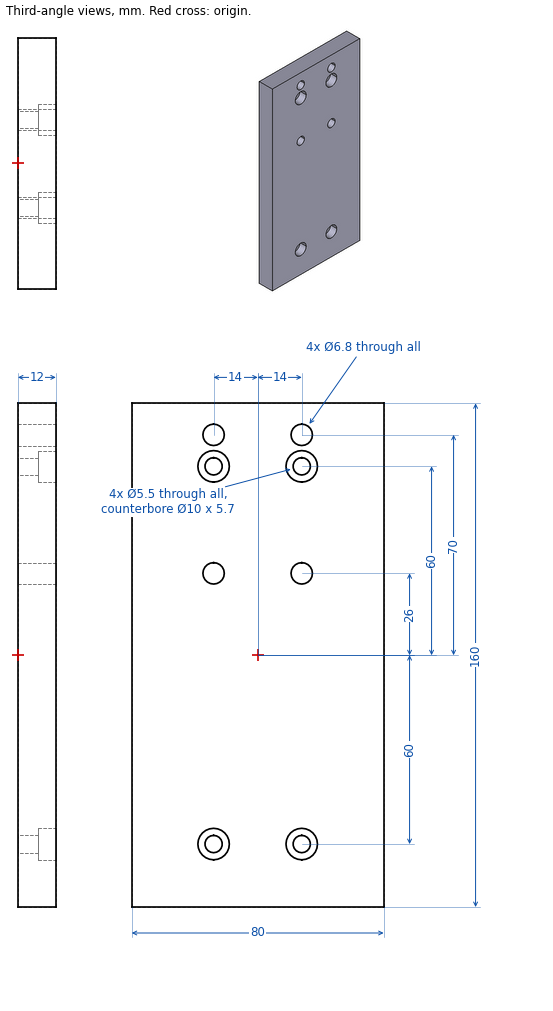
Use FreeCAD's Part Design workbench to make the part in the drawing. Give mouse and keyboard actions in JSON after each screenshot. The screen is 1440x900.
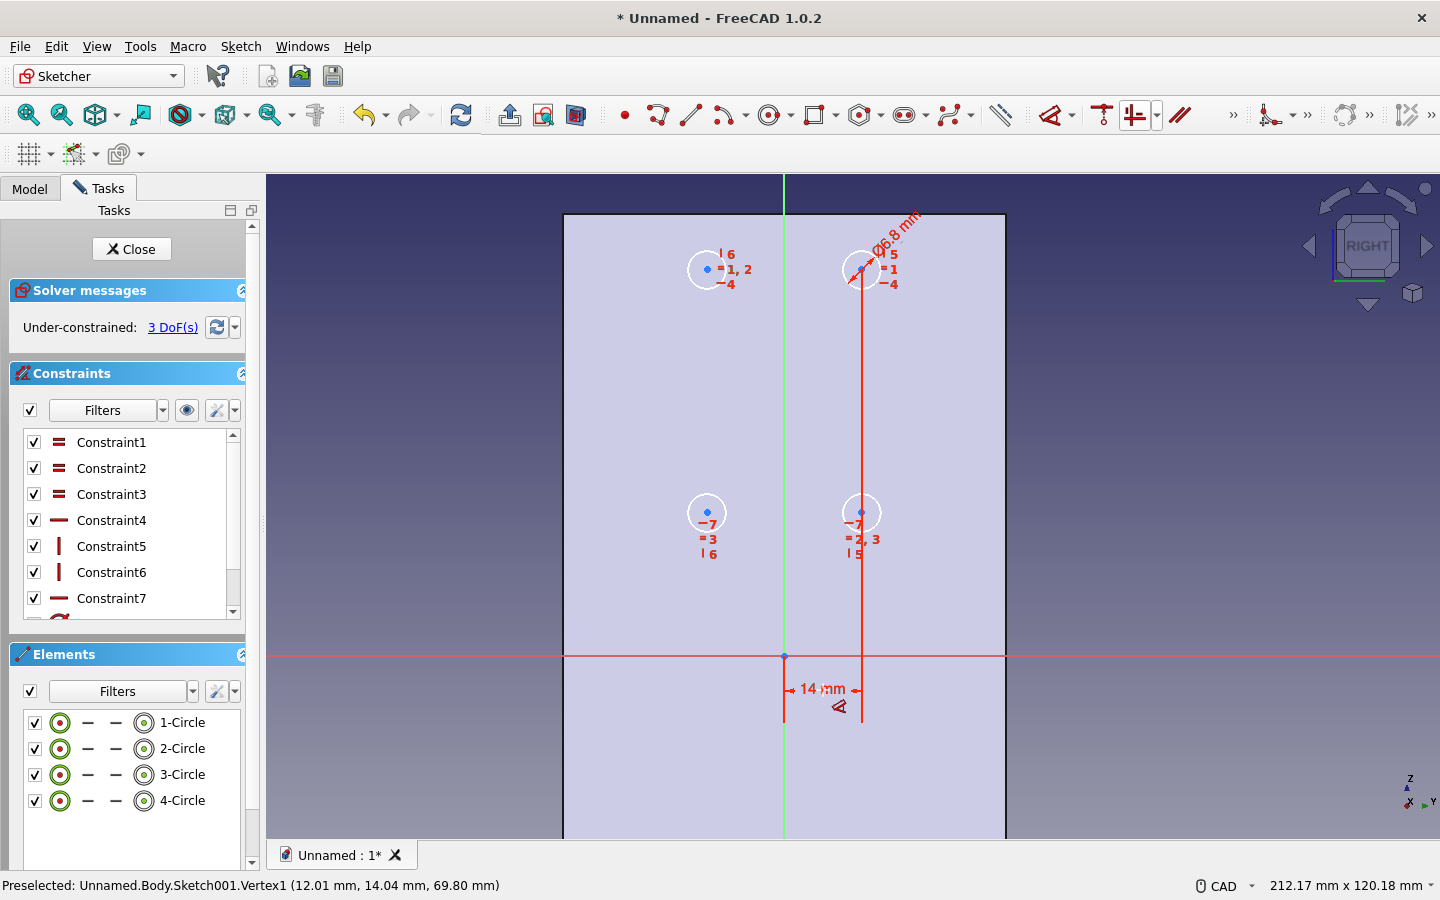
{"action": "left_click", "coordinate": [862, 270]}
{"action": "left_click", "coordinate": [896, 463]}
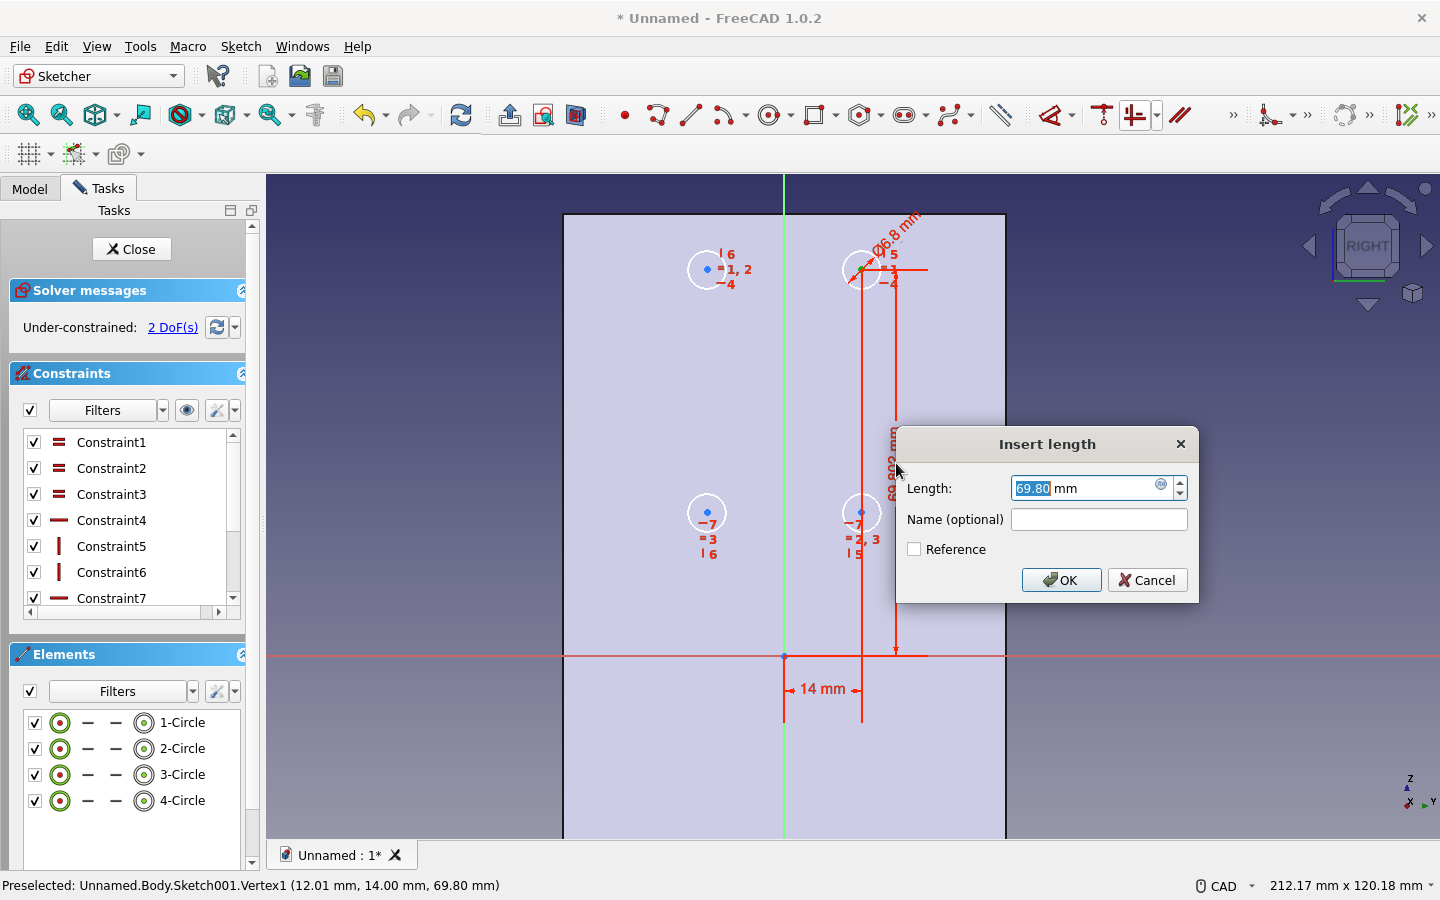
{"action": "type", "text": "70"}
{"action": "key", "text": "Return"}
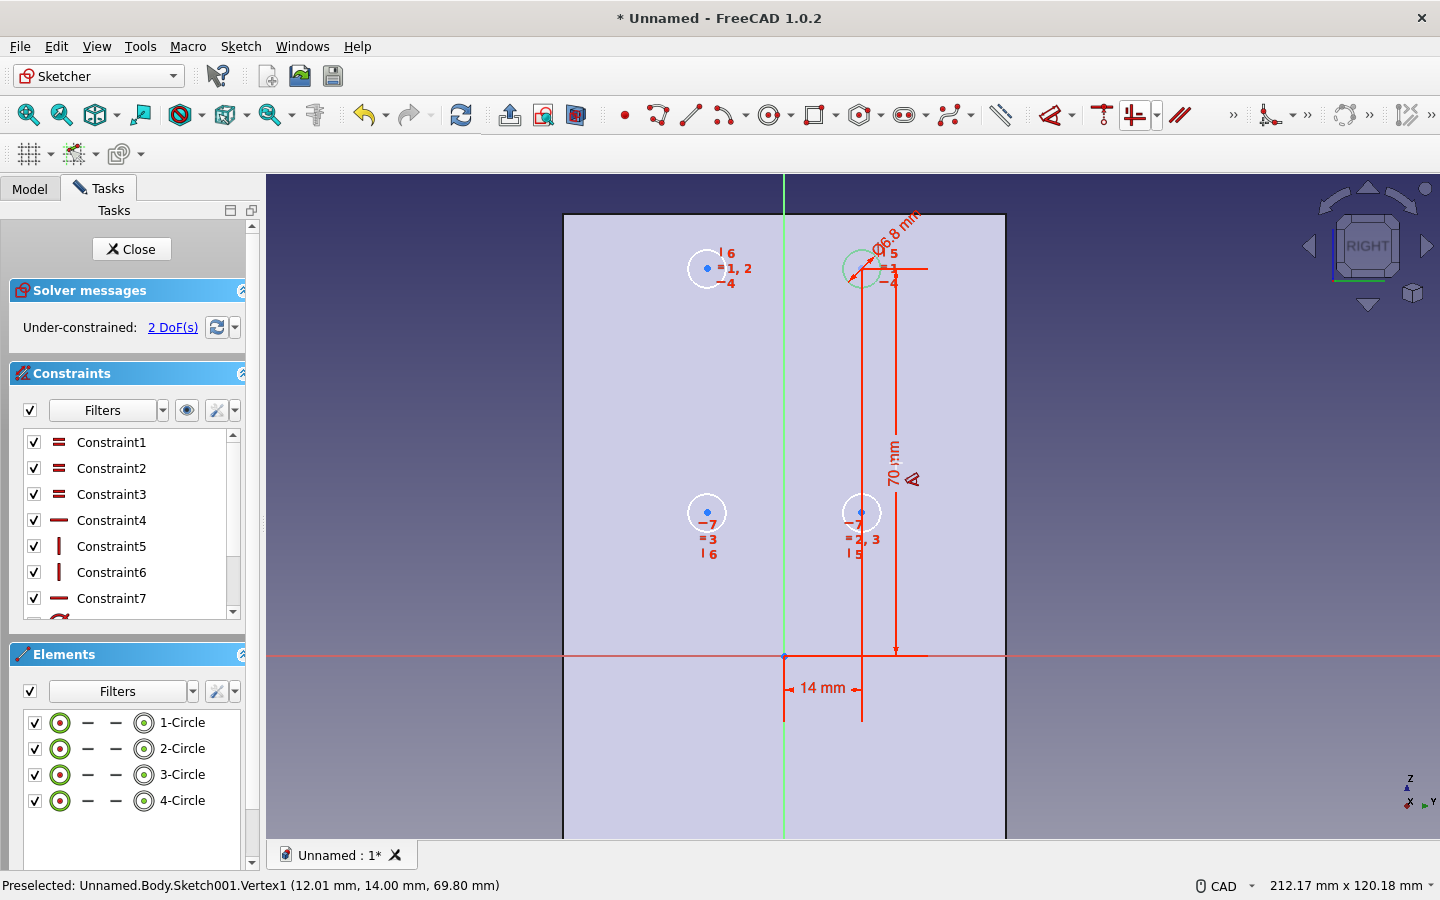
{"action": "left_click", "coordinate": [707, 269]}
{"action": "left_click", "coordinate": [746, 690]}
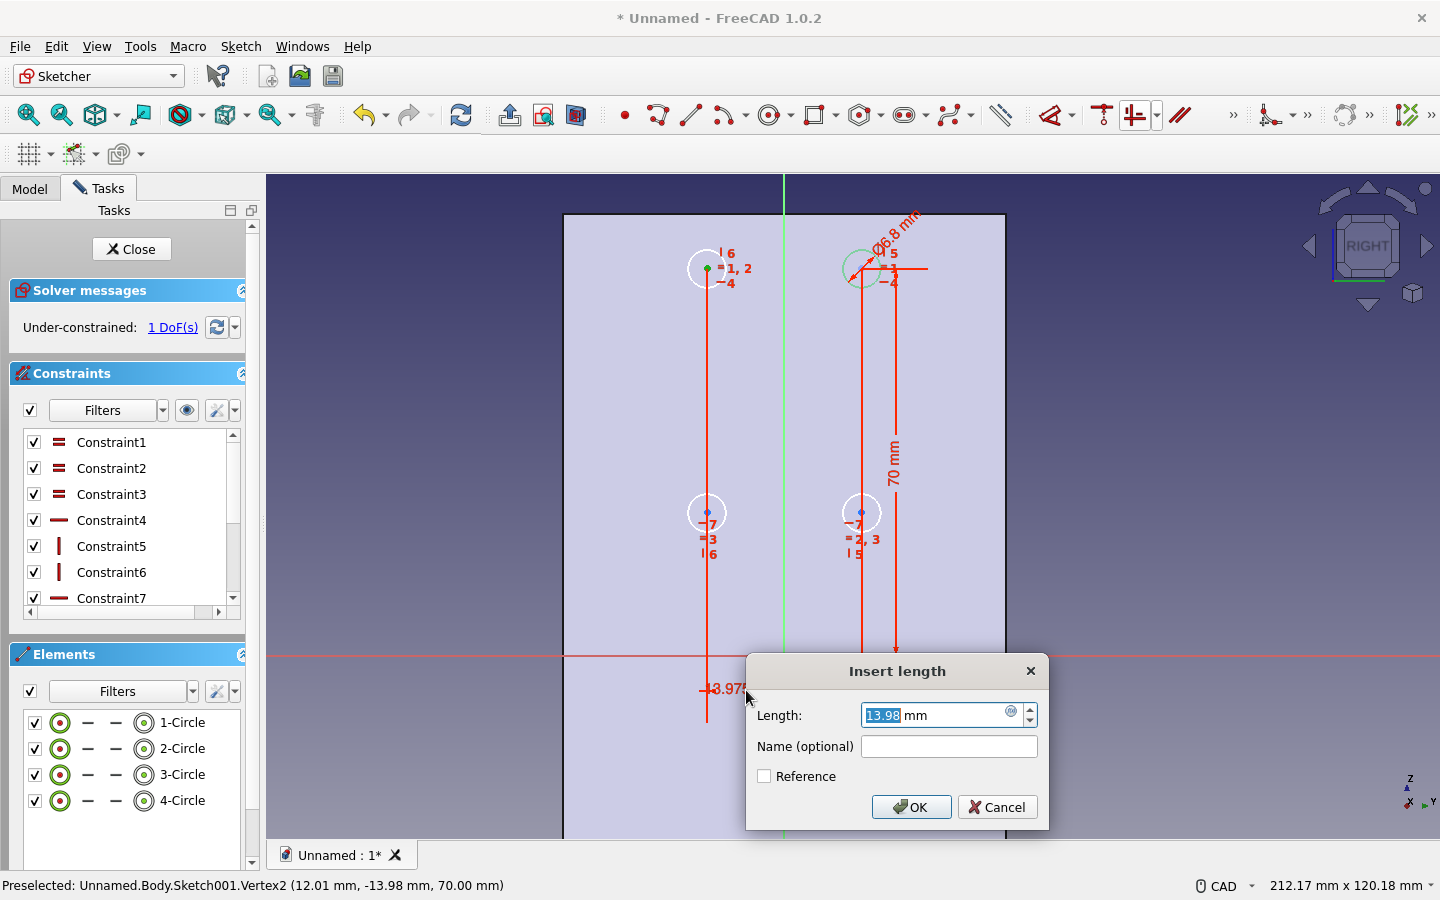
{"action": "type", "text": "14"}
{"action": "key", "text": "Return"}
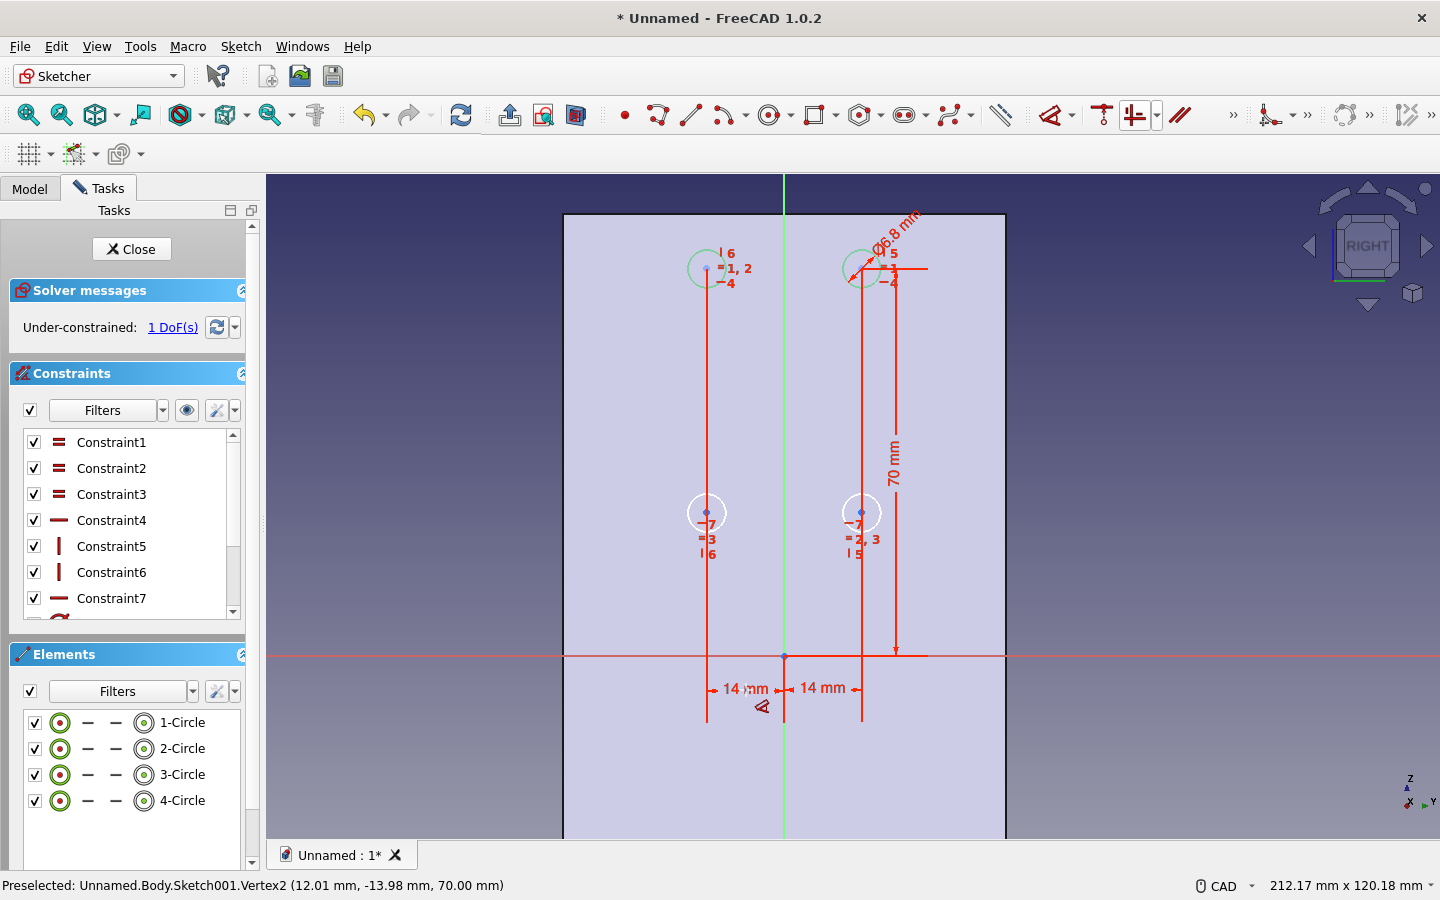
{"action": "left_click", "coordinate": [862, 513]}
{"action": "left_click", "coordinate": [896, 585]}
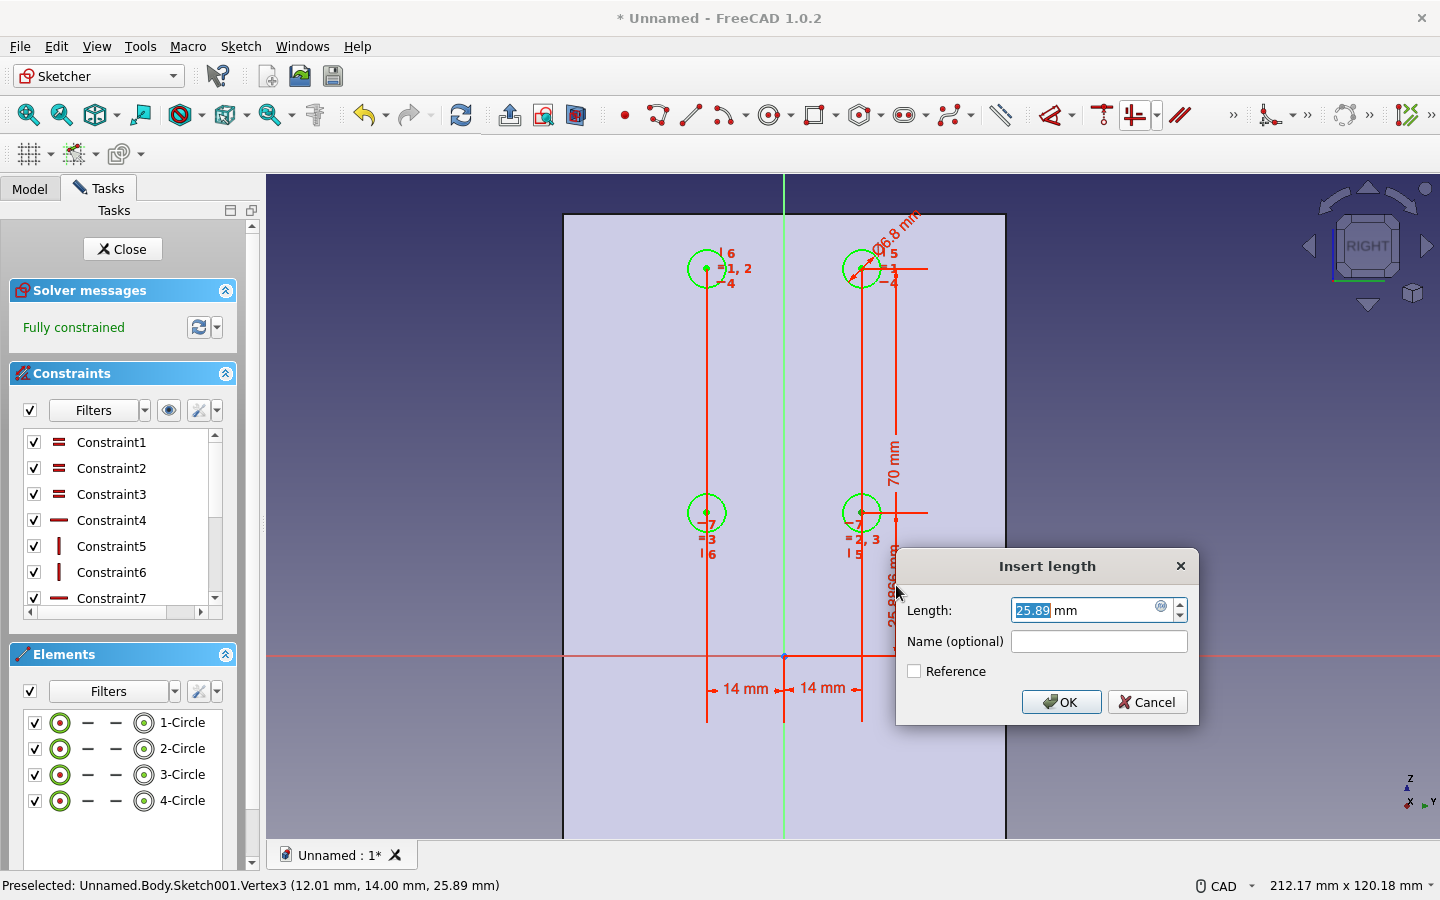
{"action": "type", "text": "26"}
{"action": "key", "text": "Return"}
{"action": "key", "text": "Escape"}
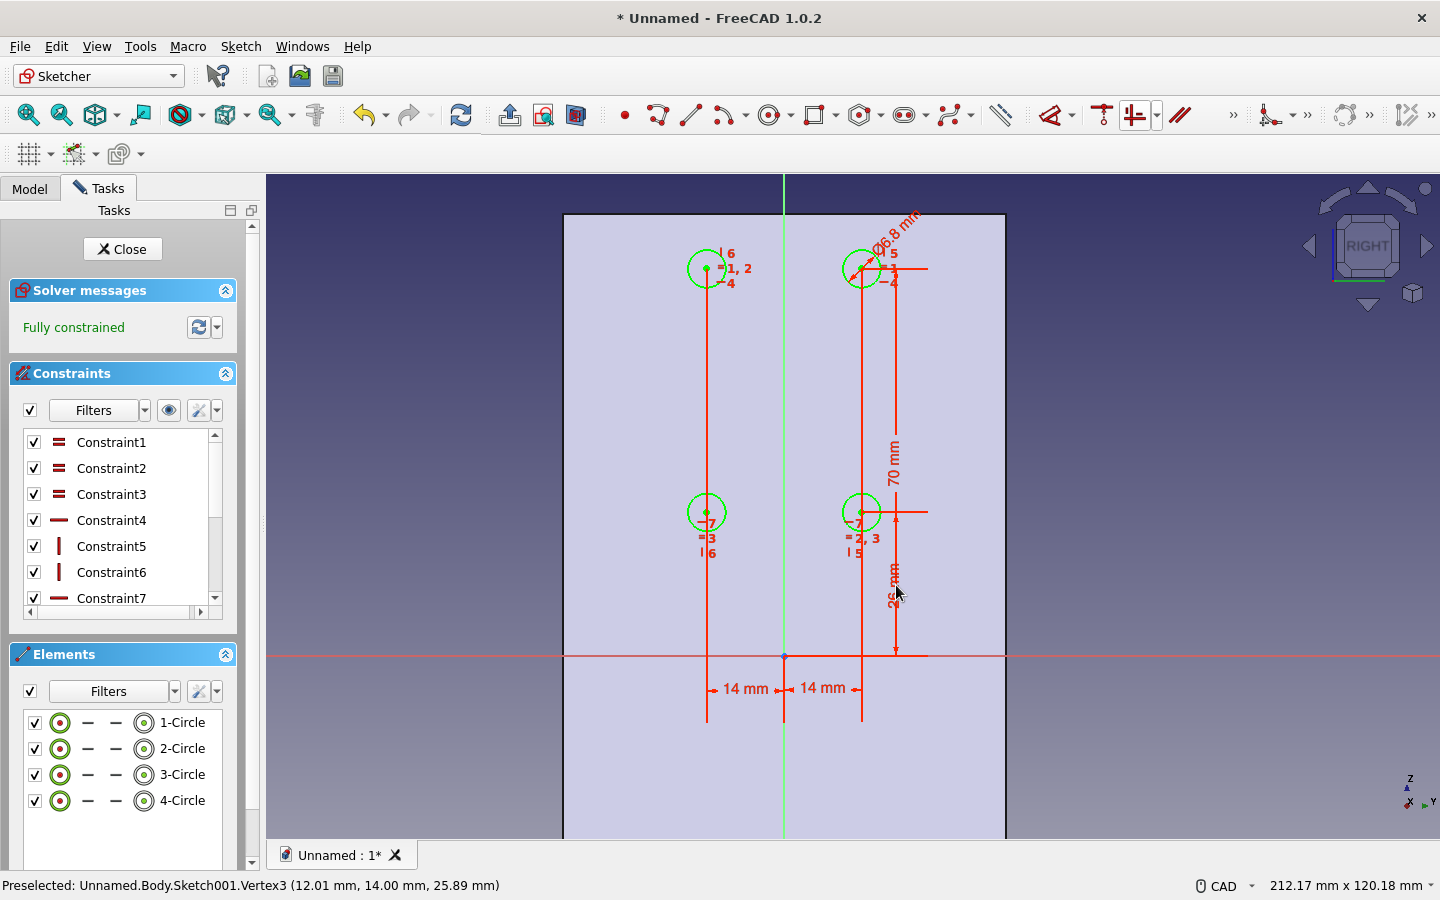
{"action": "left_click", "coordinate": [123, 249]}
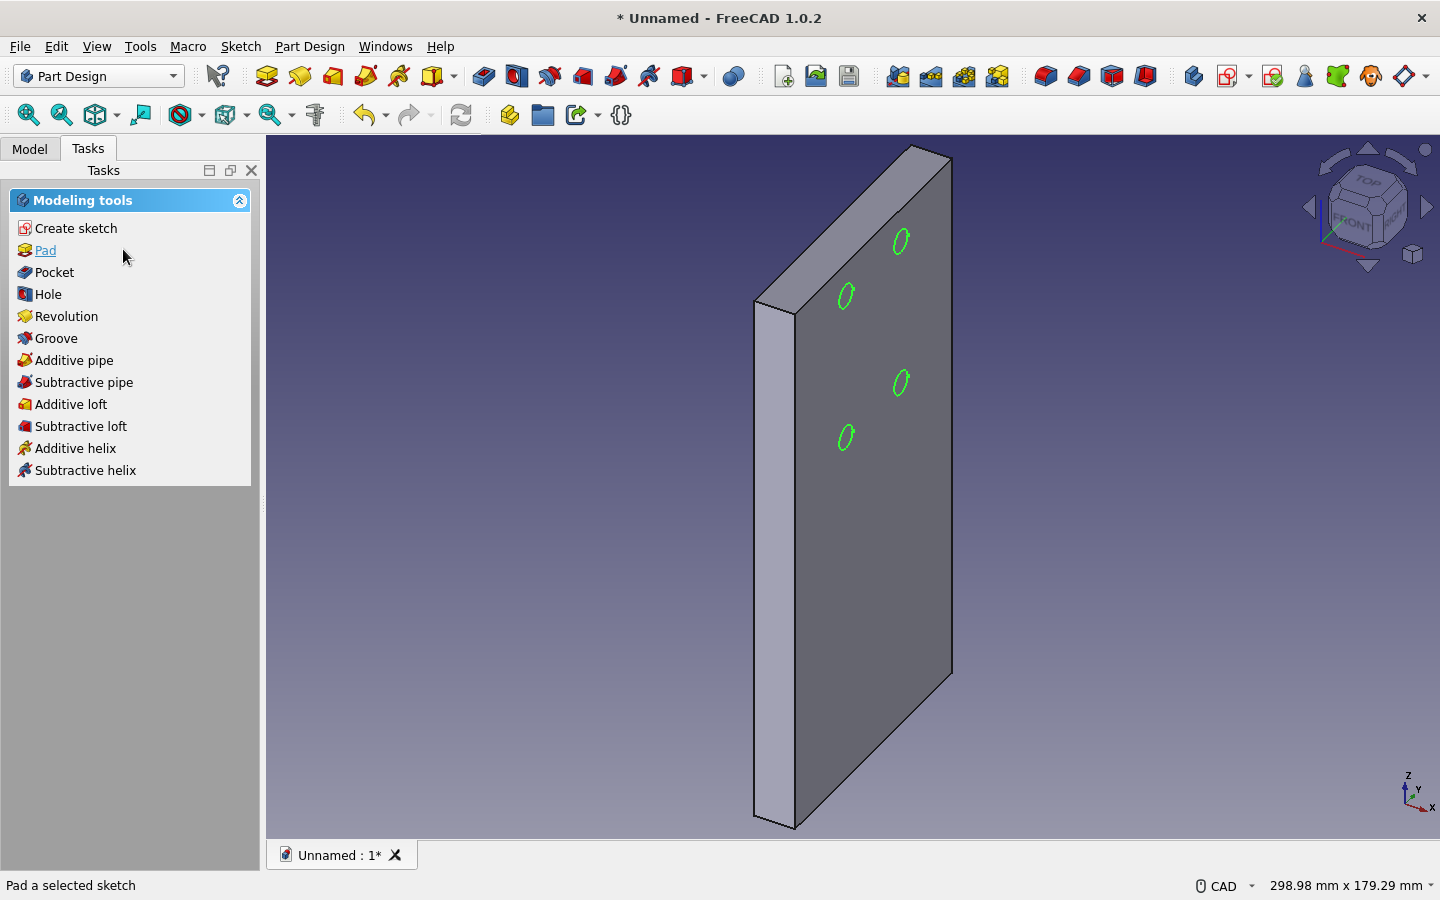
{"action": "left_click", "coordinate": [517, 76]}